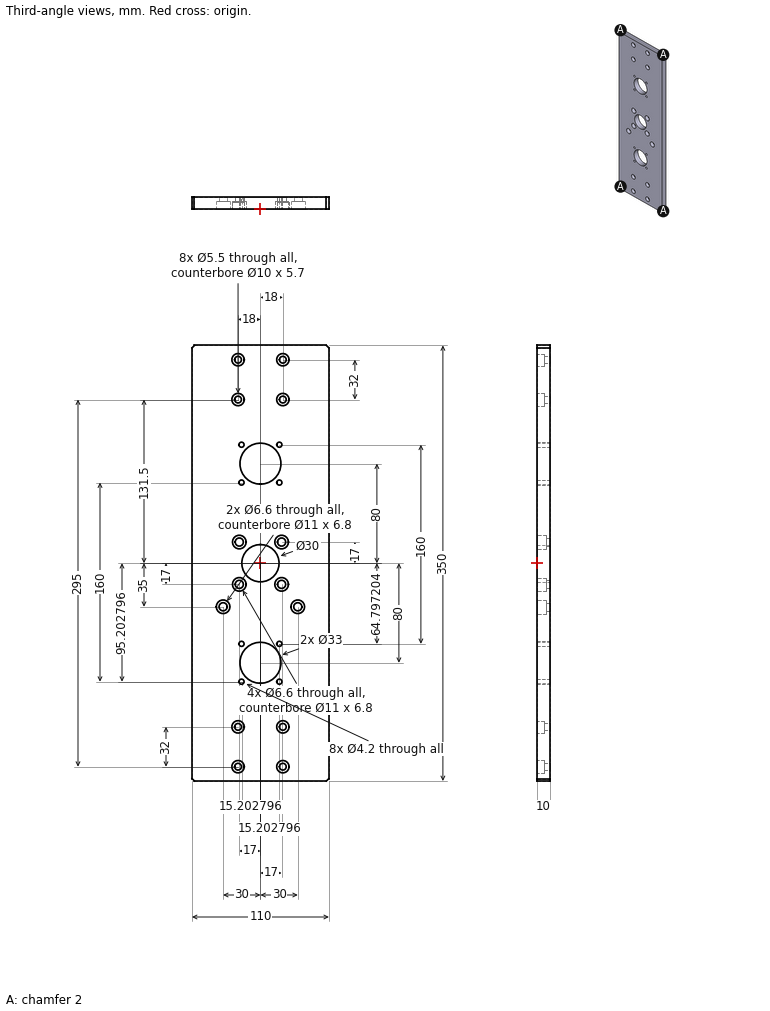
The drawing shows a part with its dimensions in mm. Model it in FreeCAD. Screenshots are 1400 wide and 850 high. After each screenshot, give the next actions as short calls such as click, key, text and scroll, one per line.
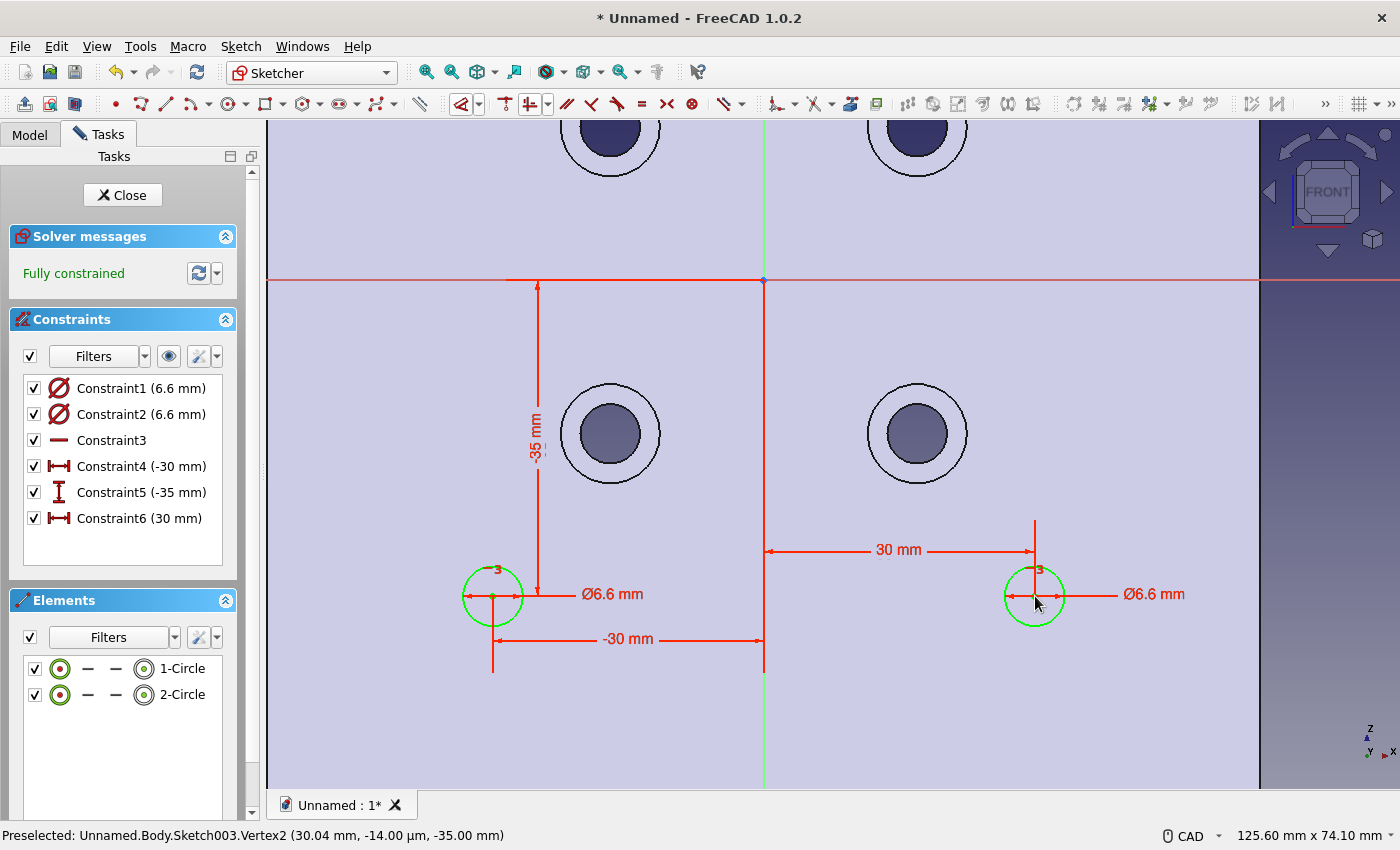
click(123, 195)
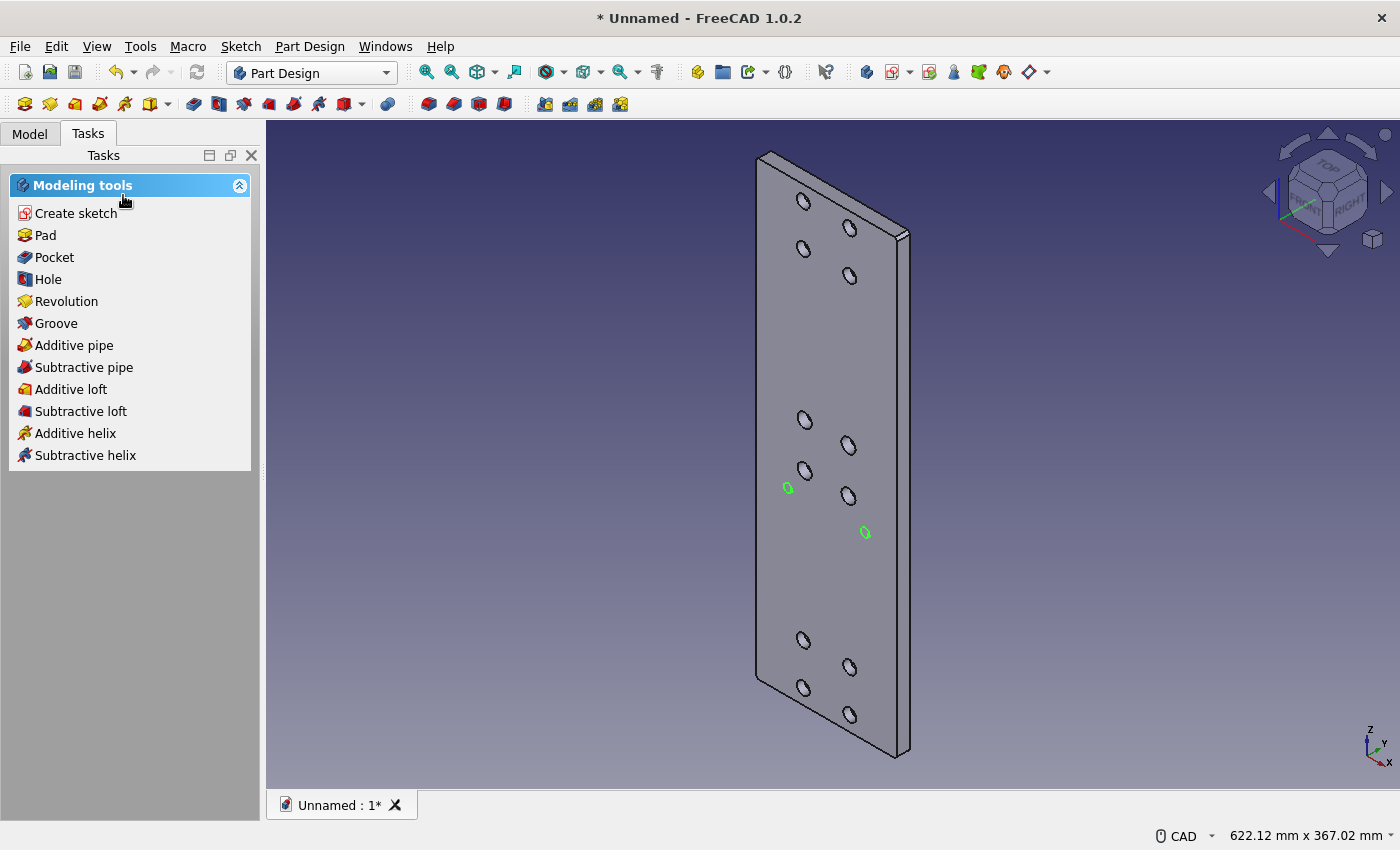
click(219, 104)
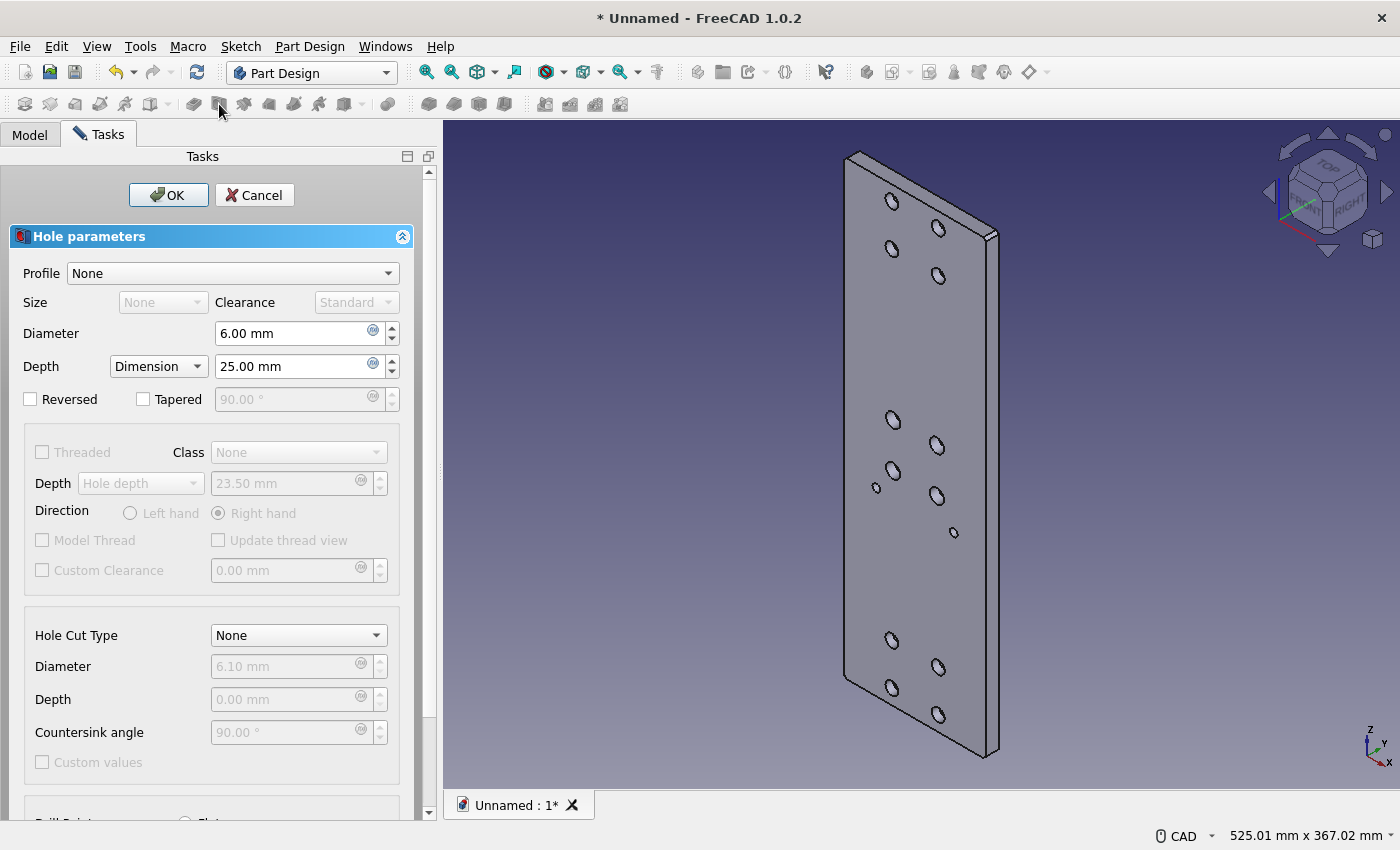
triple_click(300, 334)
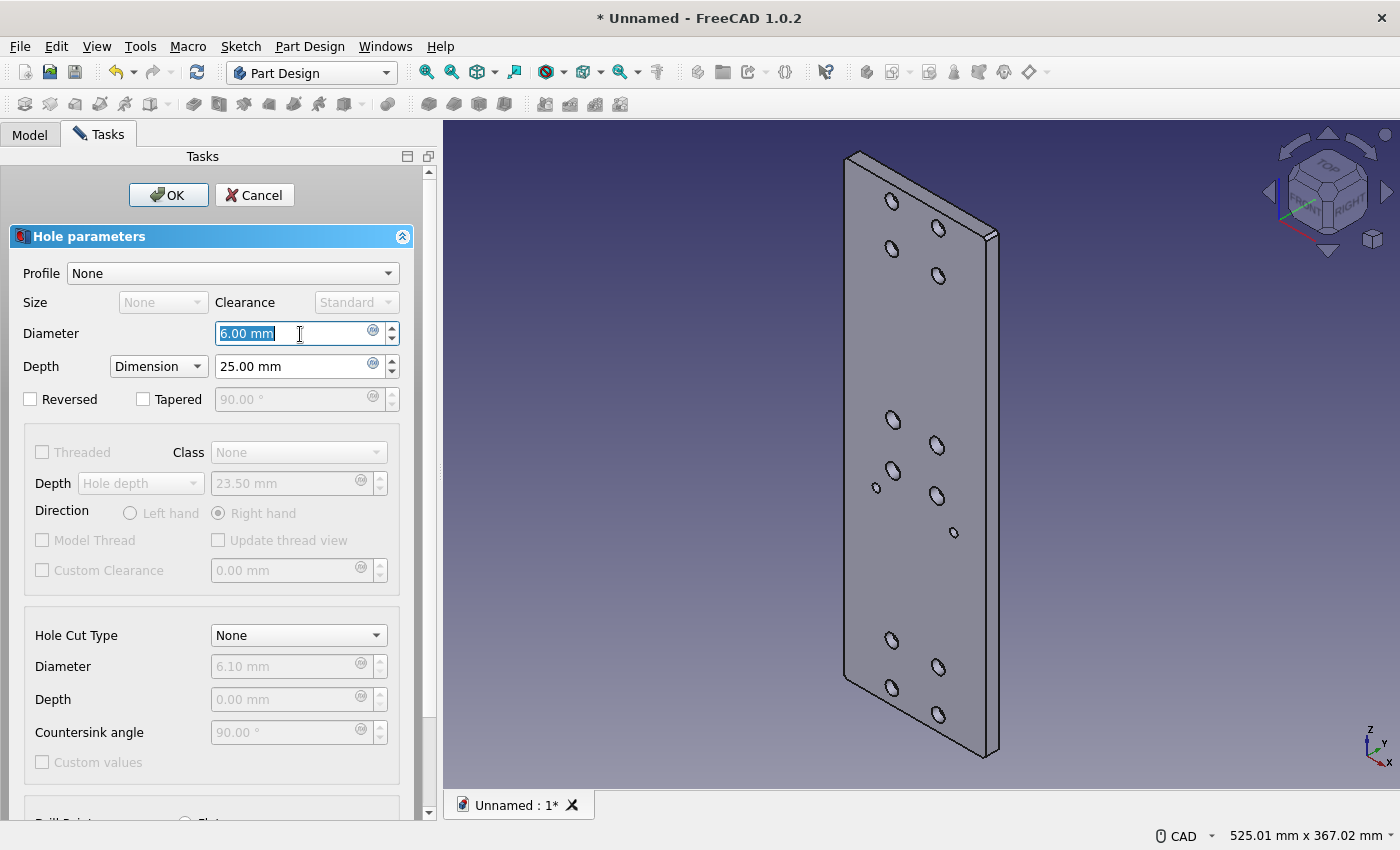
text(6.6)
key(Tab)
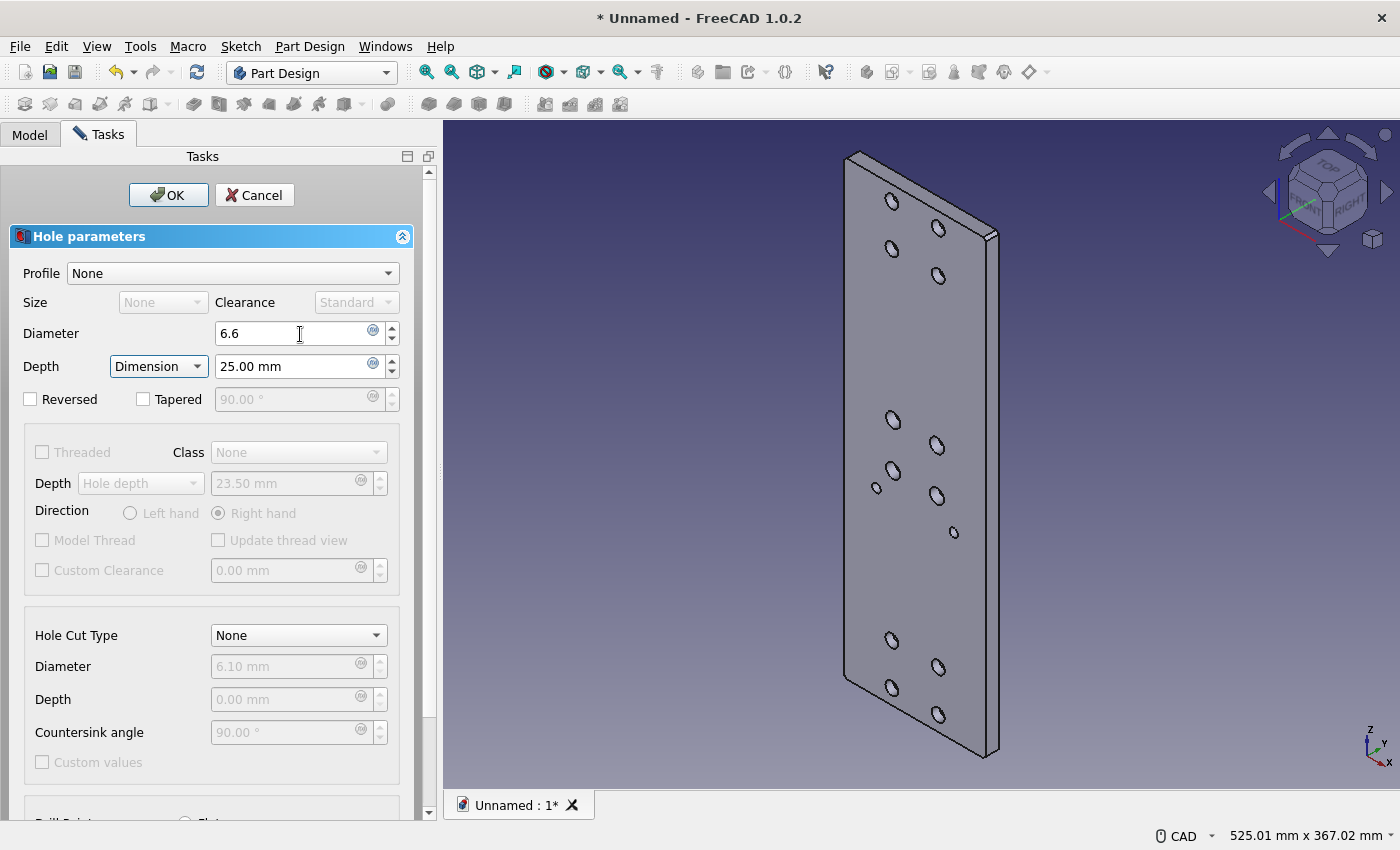
click(160, 366)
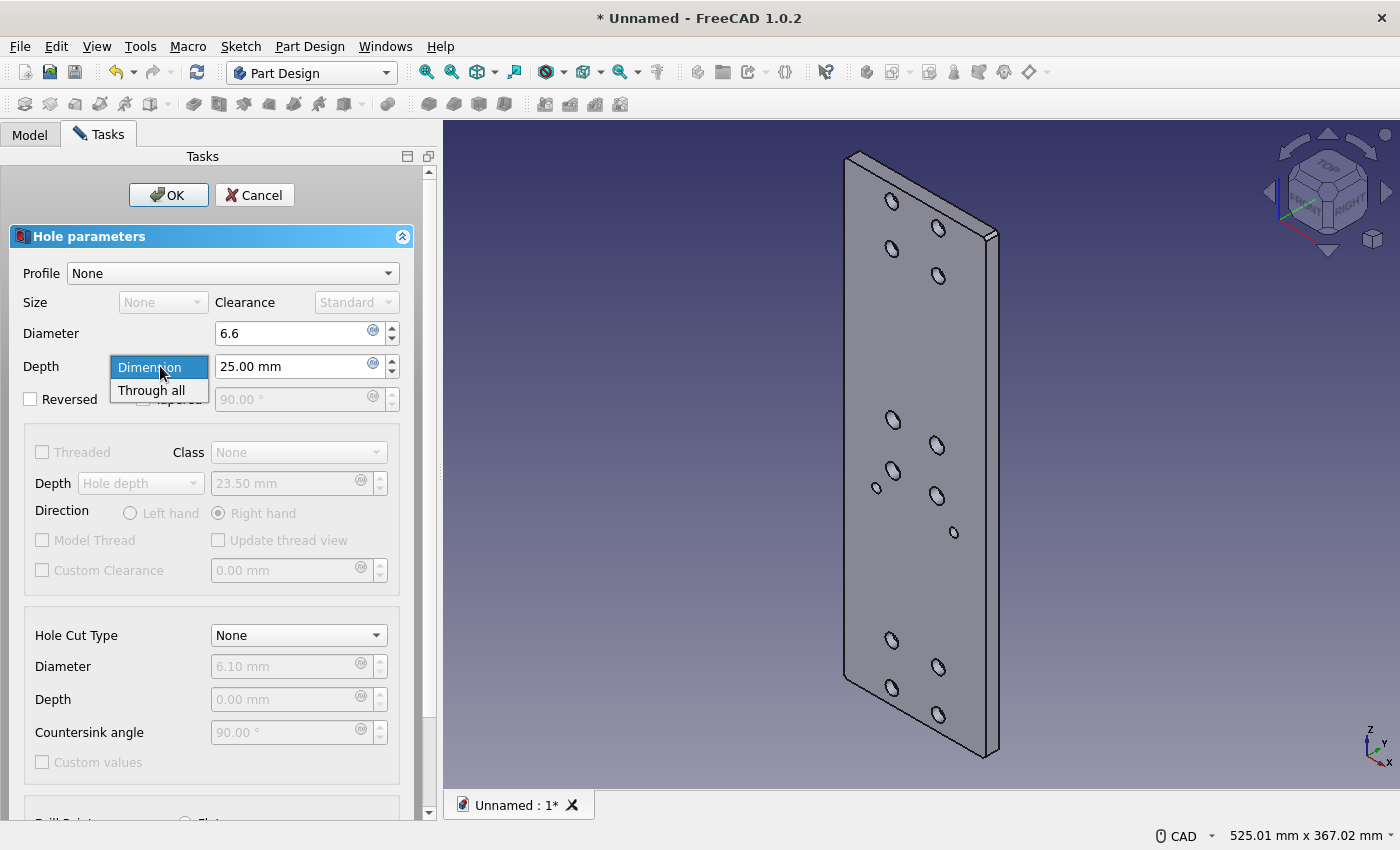
click(158, 390)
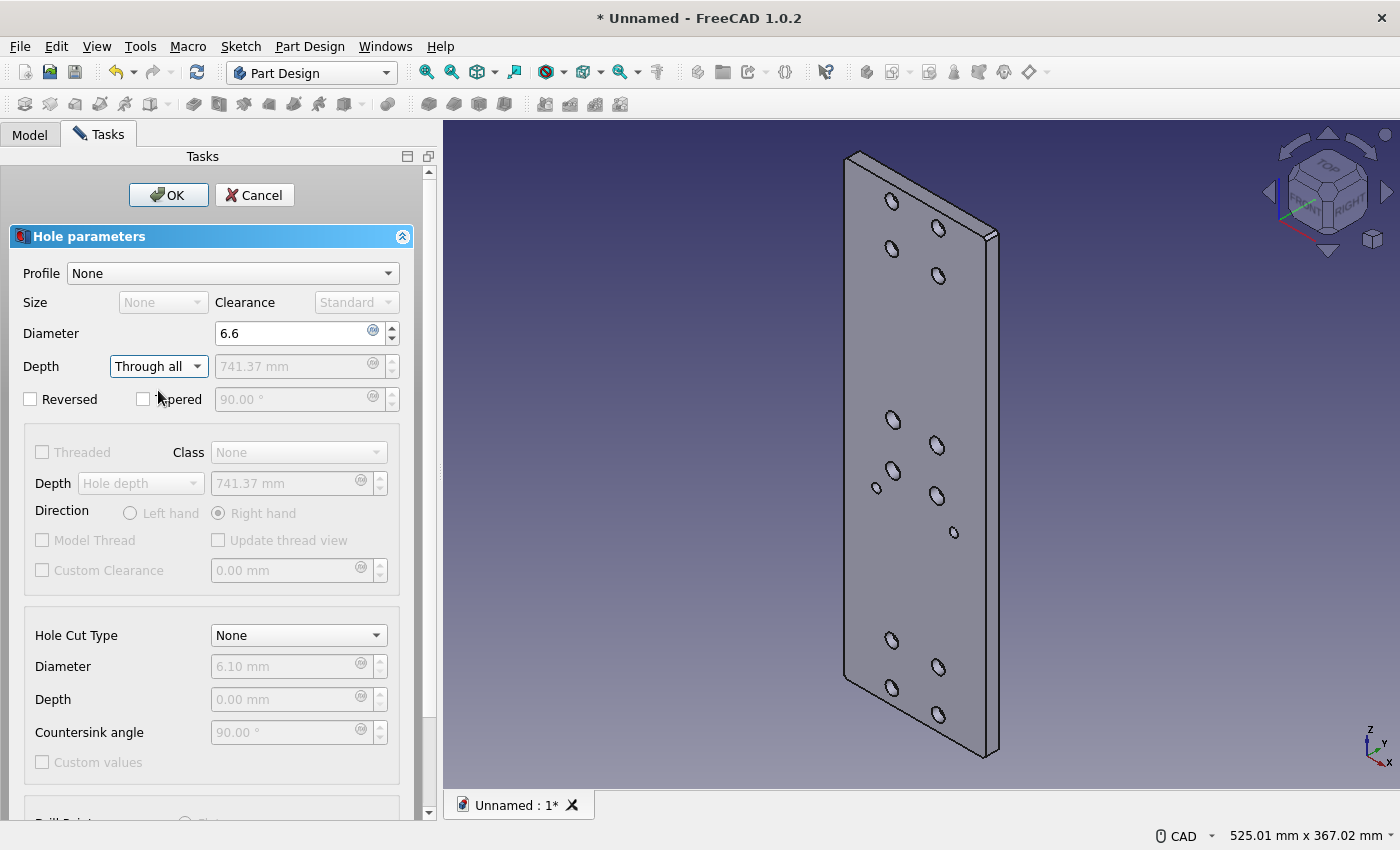
click(300, 636)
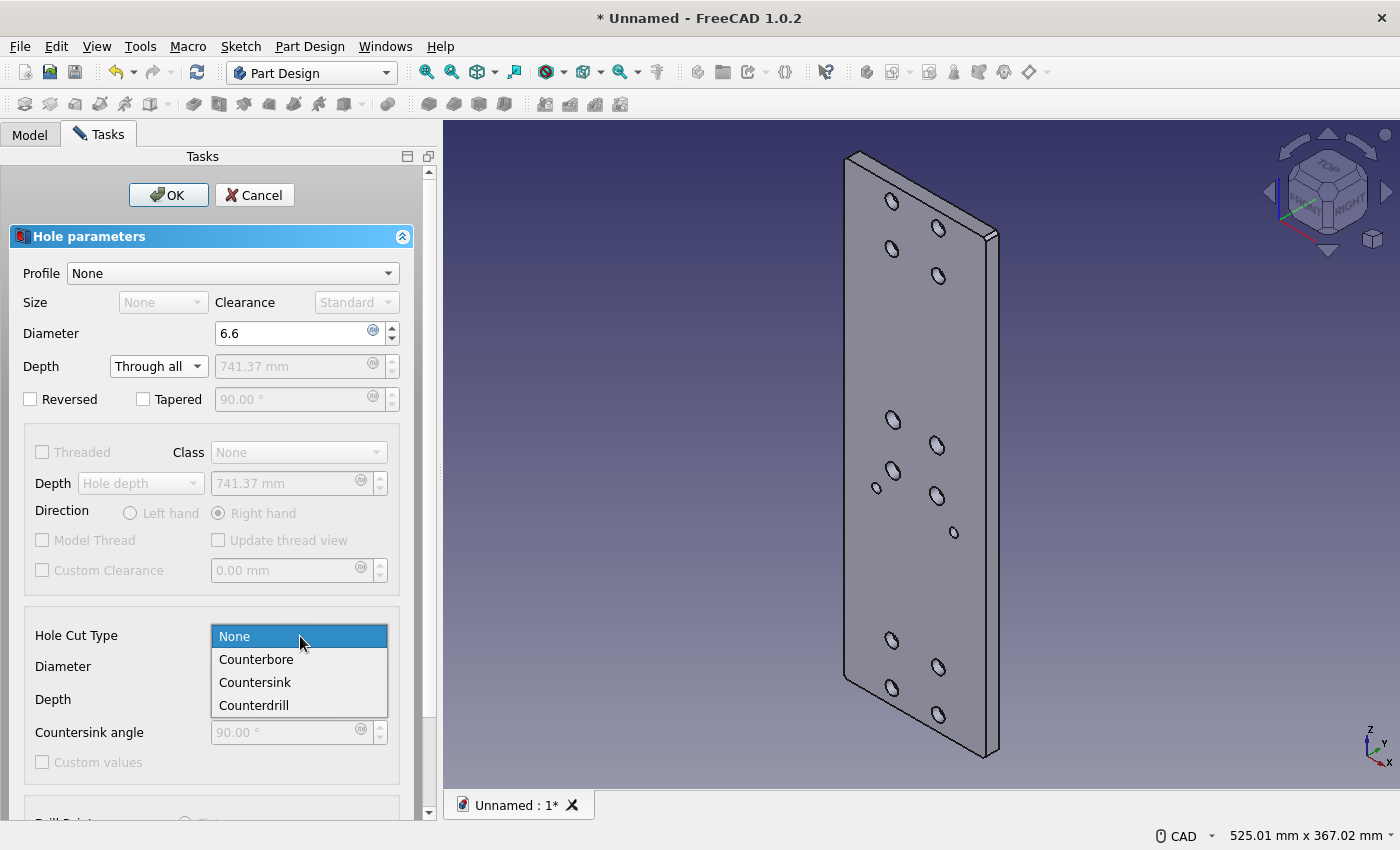
click(298, 660)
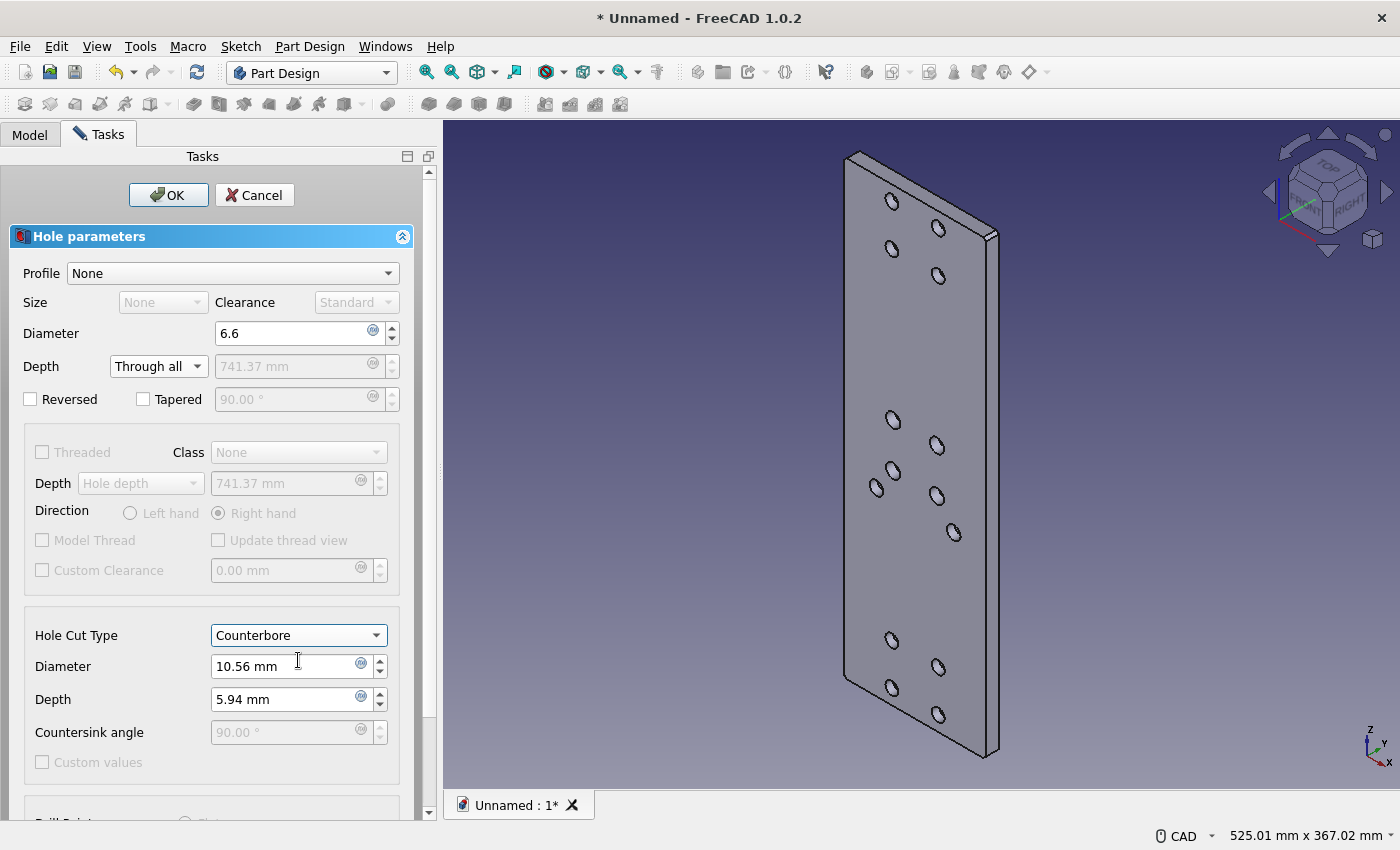
triple_click(292, 666)